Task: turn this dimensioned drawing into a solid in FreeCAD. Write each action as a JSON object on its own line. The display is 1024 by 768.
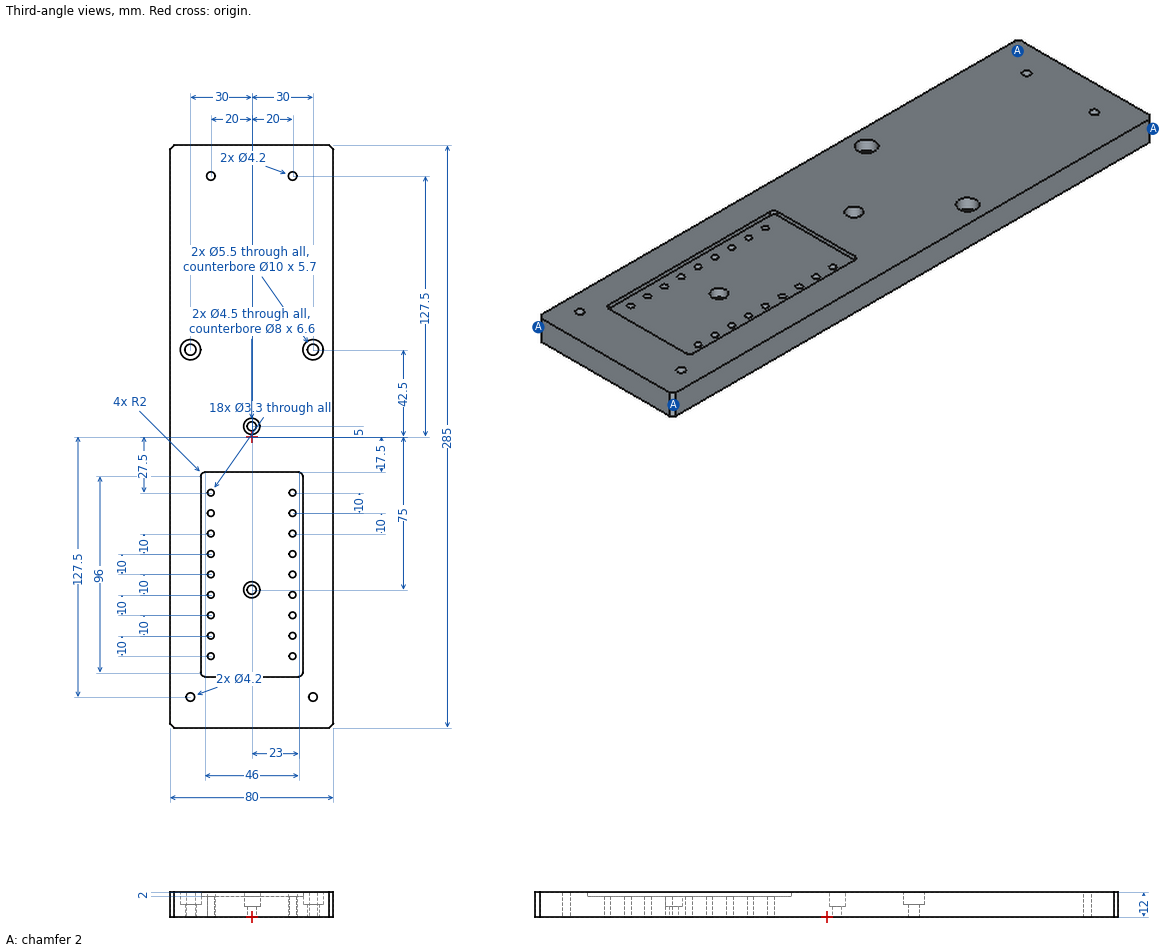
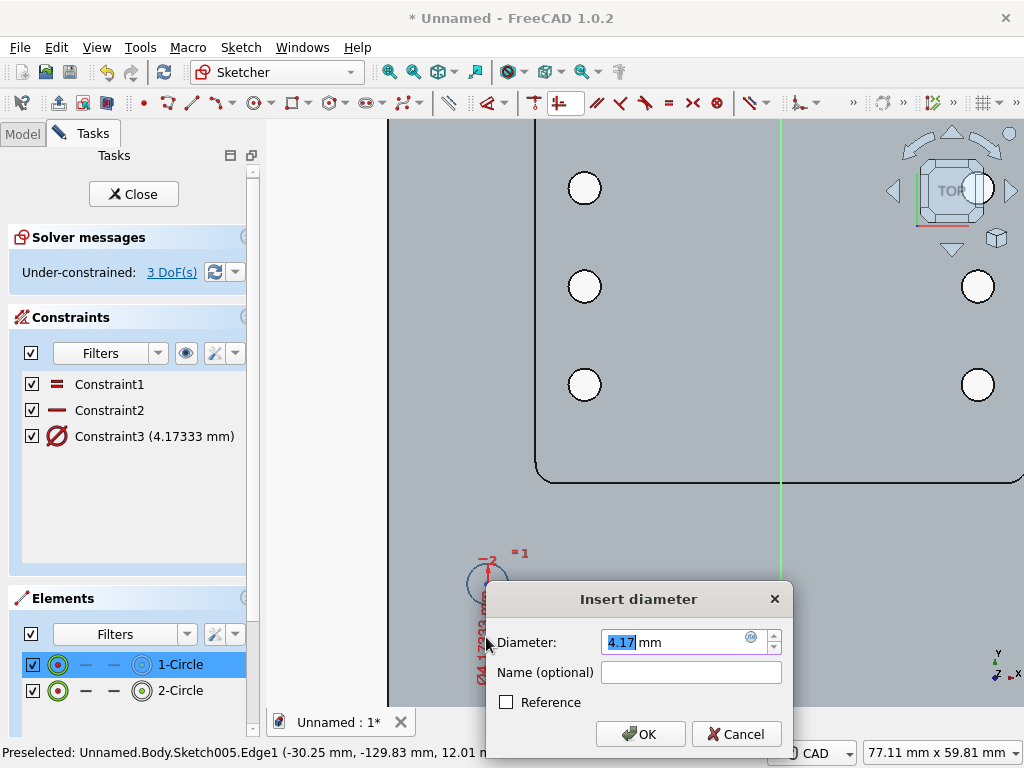
{"action": "type", "text": "4.2"}
{"action": "key", "text": "Return"}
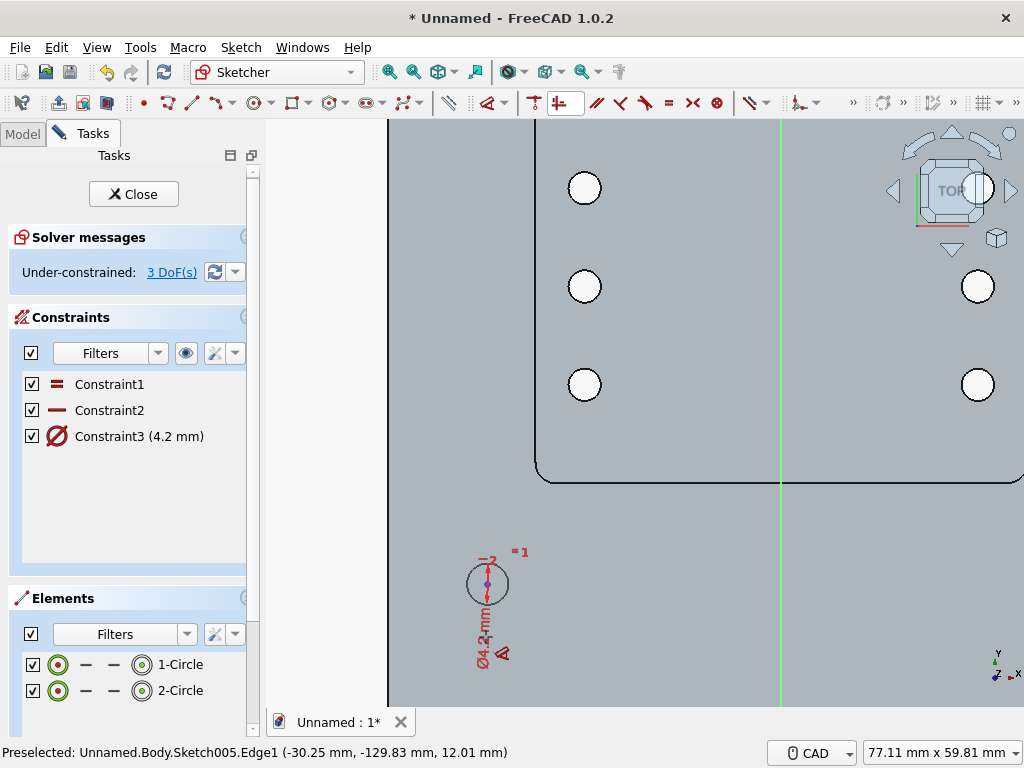
{"action": "left_click", "coordinate": [488, 584]}
{"action": "left_click", "coordinate": [634, 618]}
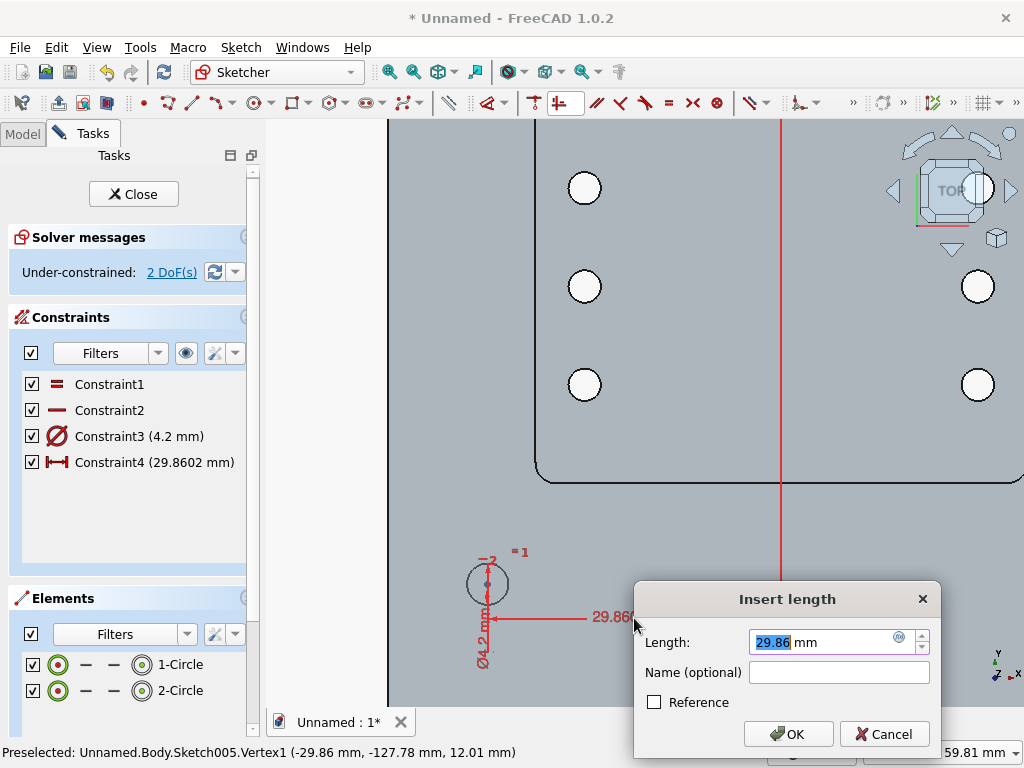
{"action": "type", "text": "30"}
{"action": "key", "text": "Return"}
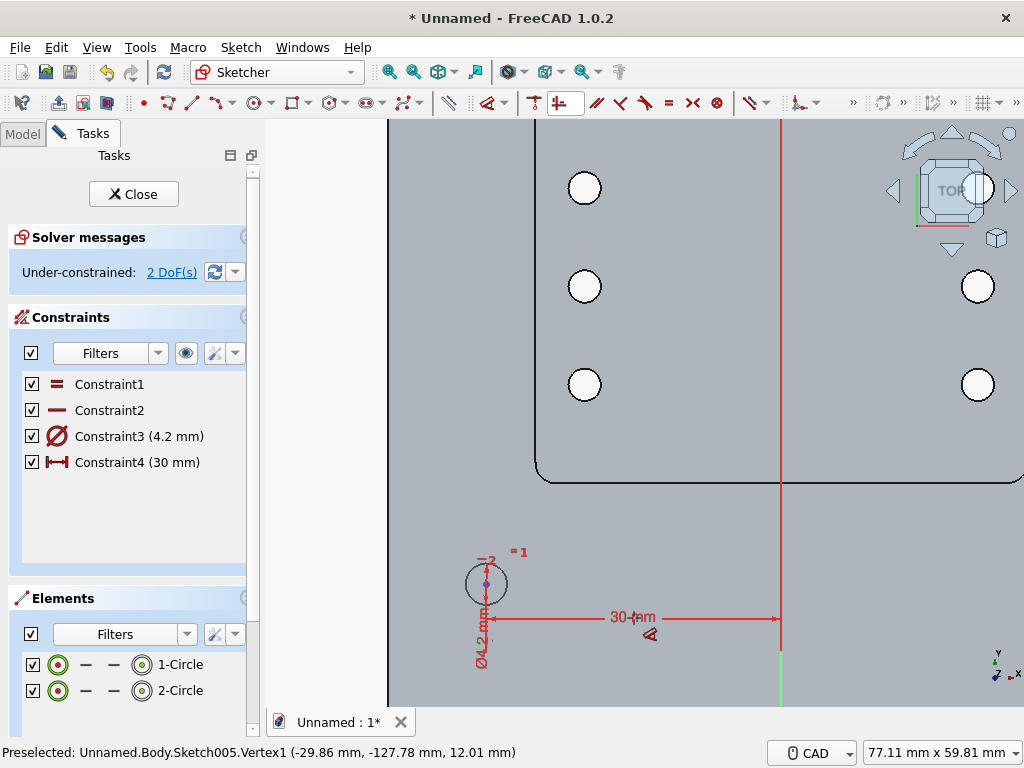
{"action": "scroll", "coordinate": [488, 606], "scroll_direction": "down", "scroll_amount": 6}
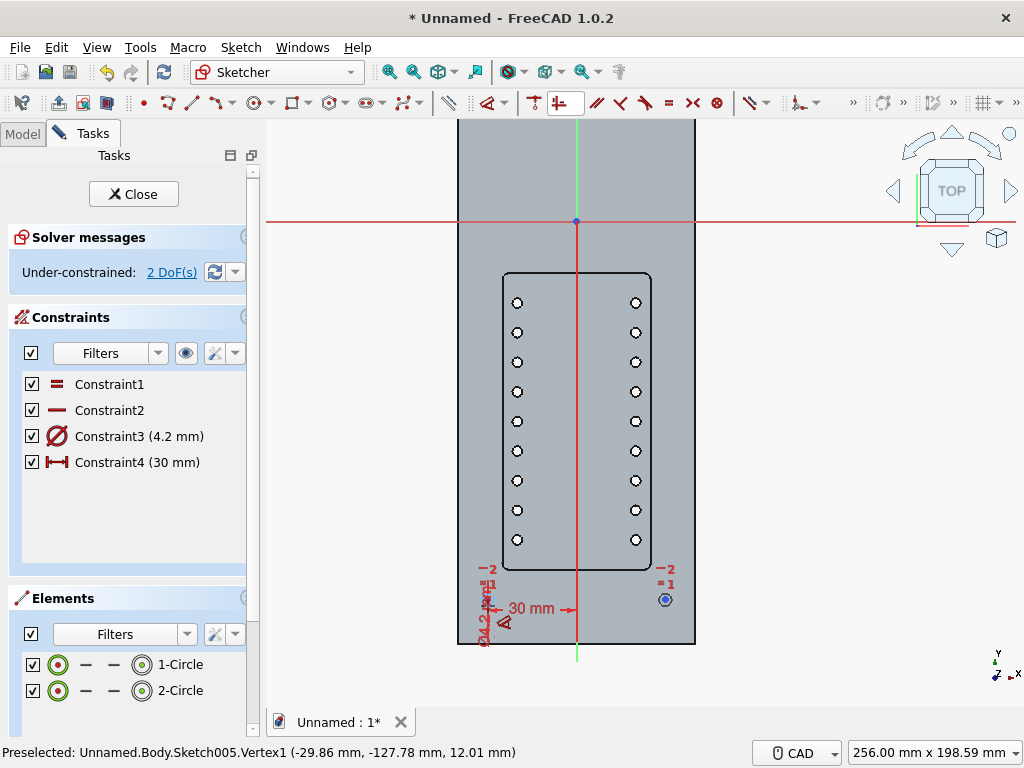
{"action": "left_click", "coordinate": [665, 600]}
{"action": "left_click", "coordinate": [621, 188]}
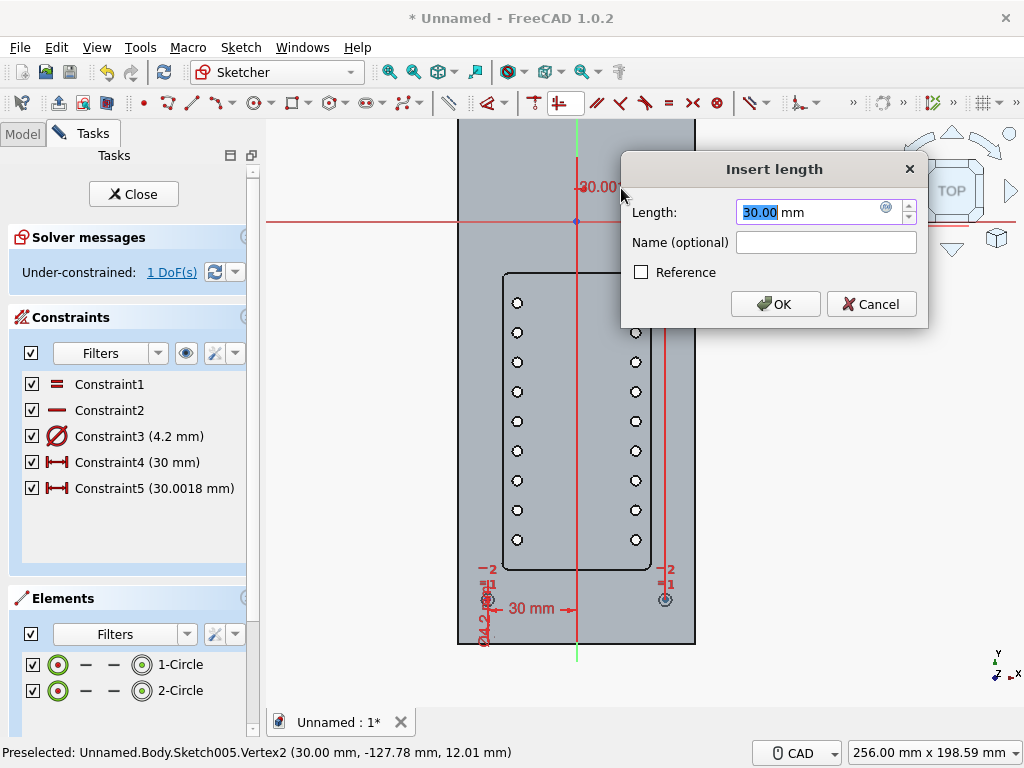
{"action": "type", "text": "30"}
{"action": "key", "text": "Return"}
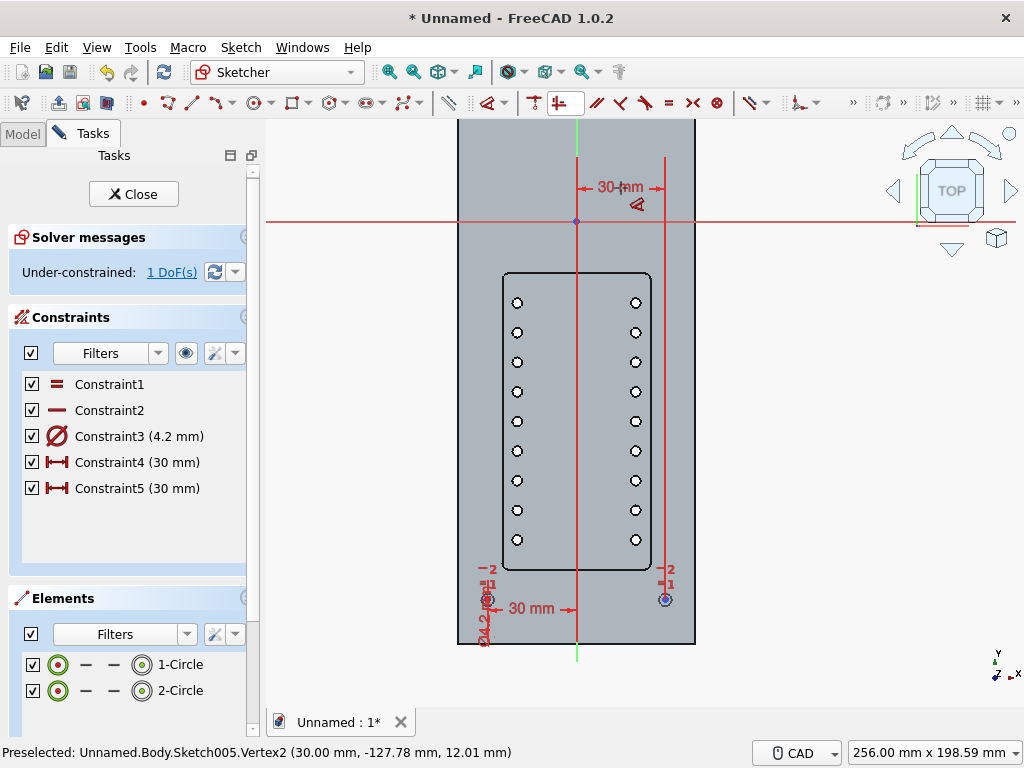
{"action": "left_click", "coordinate": [488, 600]}
{"action": "left_click", "coordinate": [454, 411]}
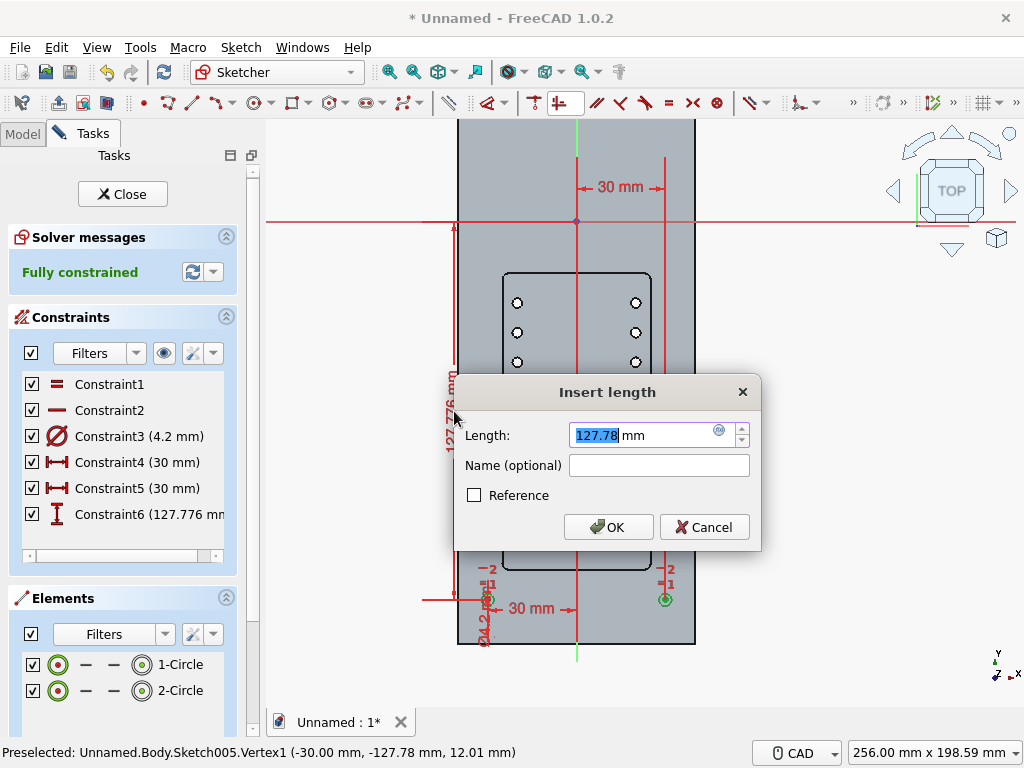
{"action": "type", "text": "127.5"}
{"action": "key", "text": "Return"}
{"action": "key", "text": "Escape"}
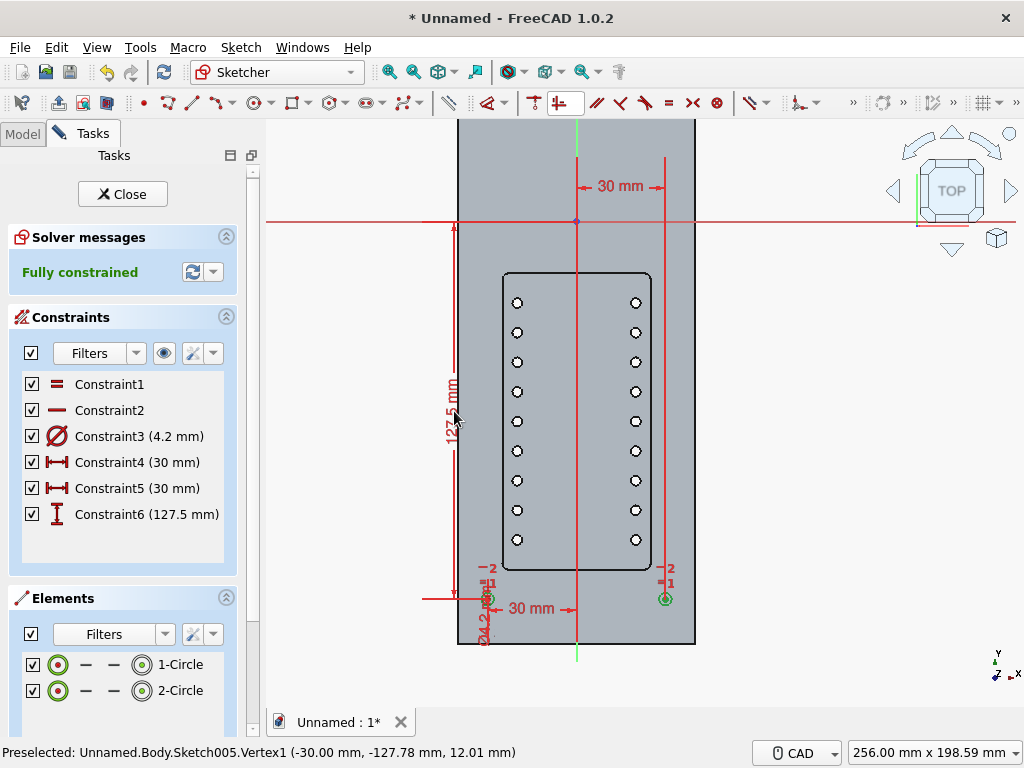
{"action": "left_click", "coordinate": [123, 194]}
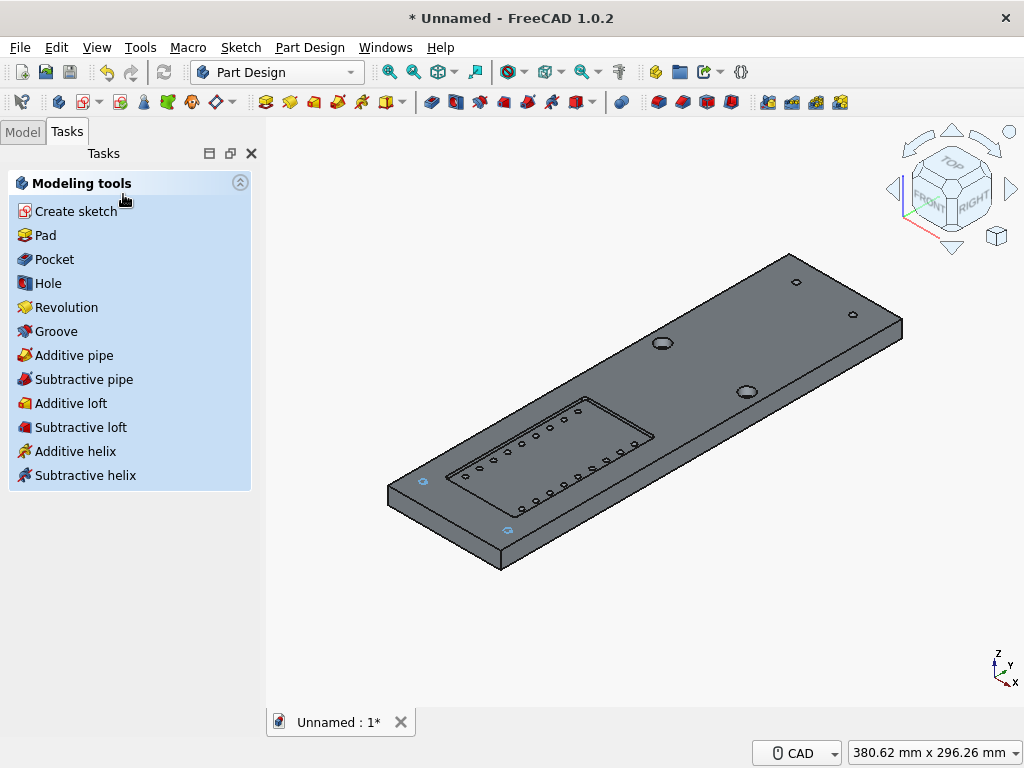
{"action": "left_click", "coordinate": [432, 102]}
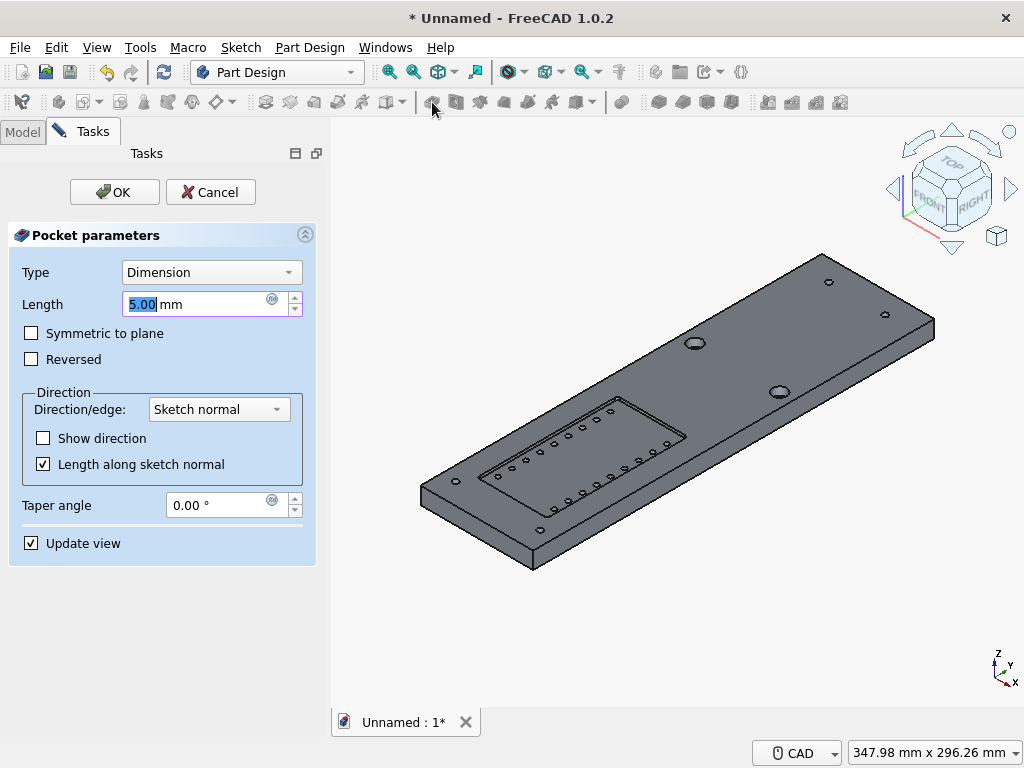
{"action": "left_click", "coordinate": [212, 272]}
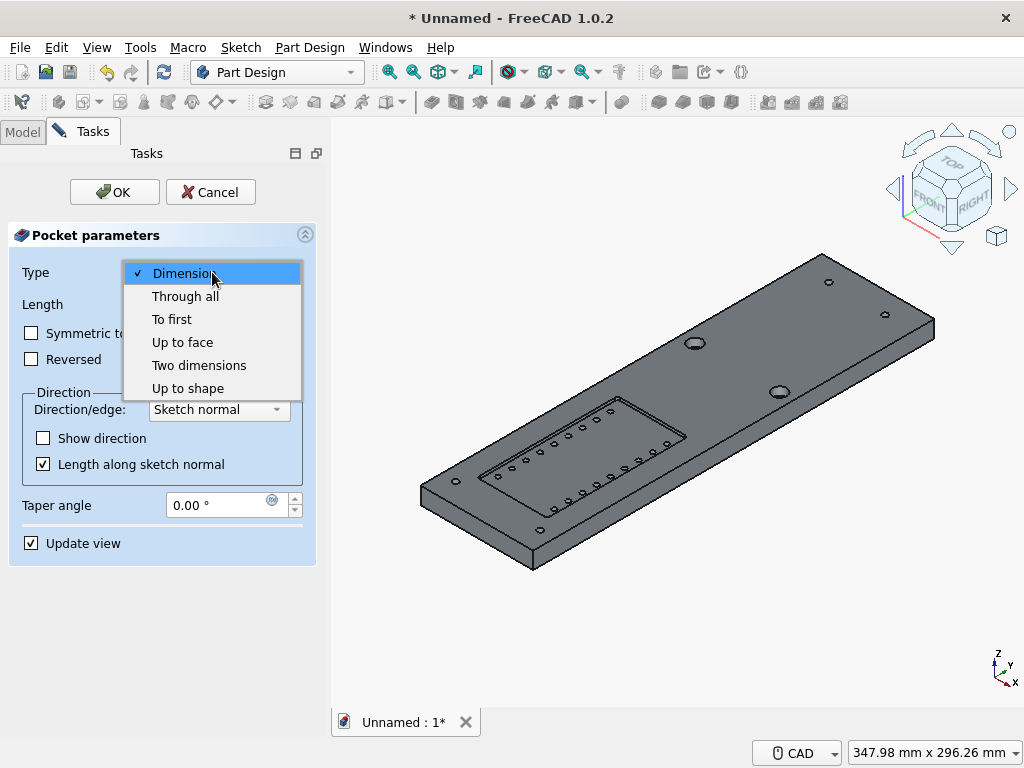
{"action": "left_click", "coordinate": [212, 296]}